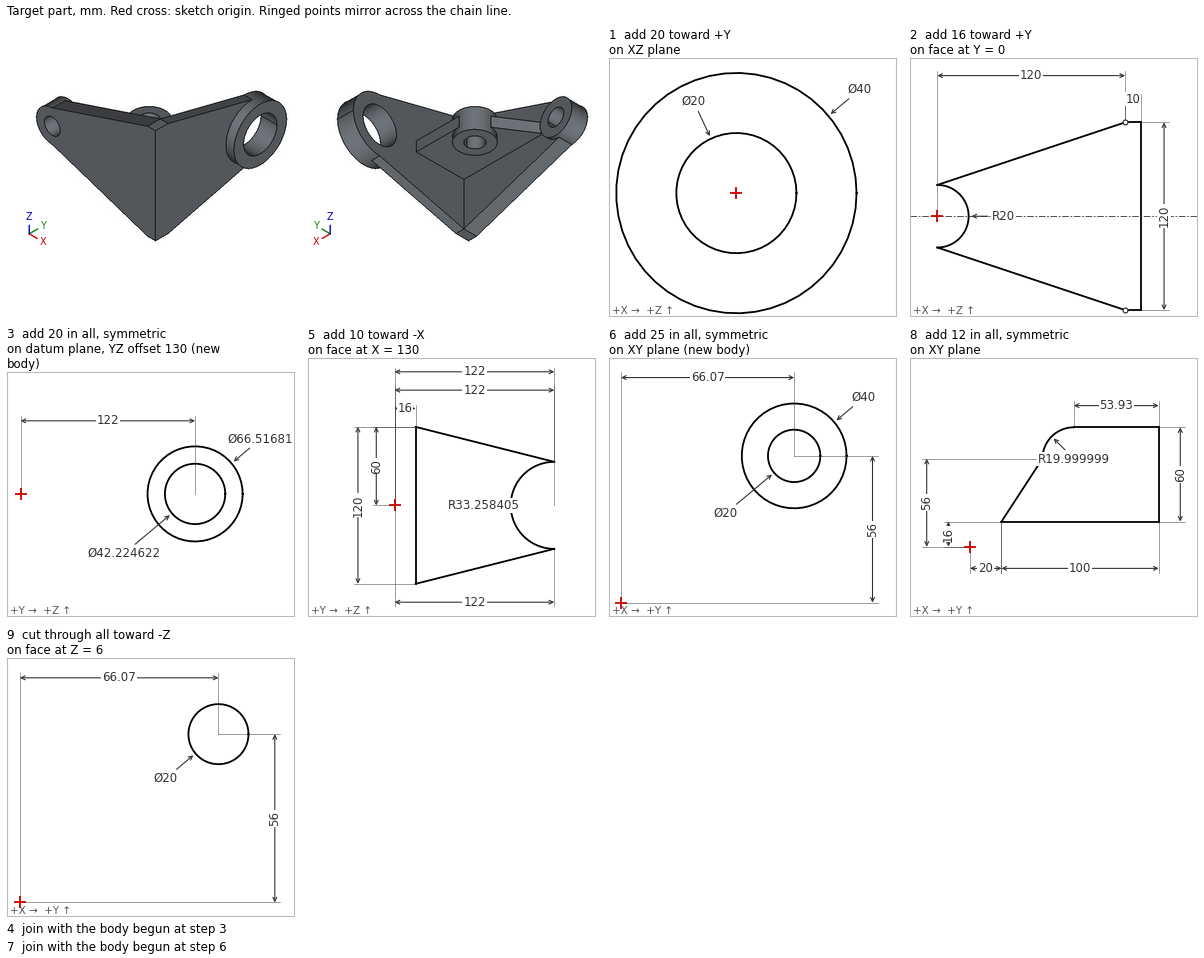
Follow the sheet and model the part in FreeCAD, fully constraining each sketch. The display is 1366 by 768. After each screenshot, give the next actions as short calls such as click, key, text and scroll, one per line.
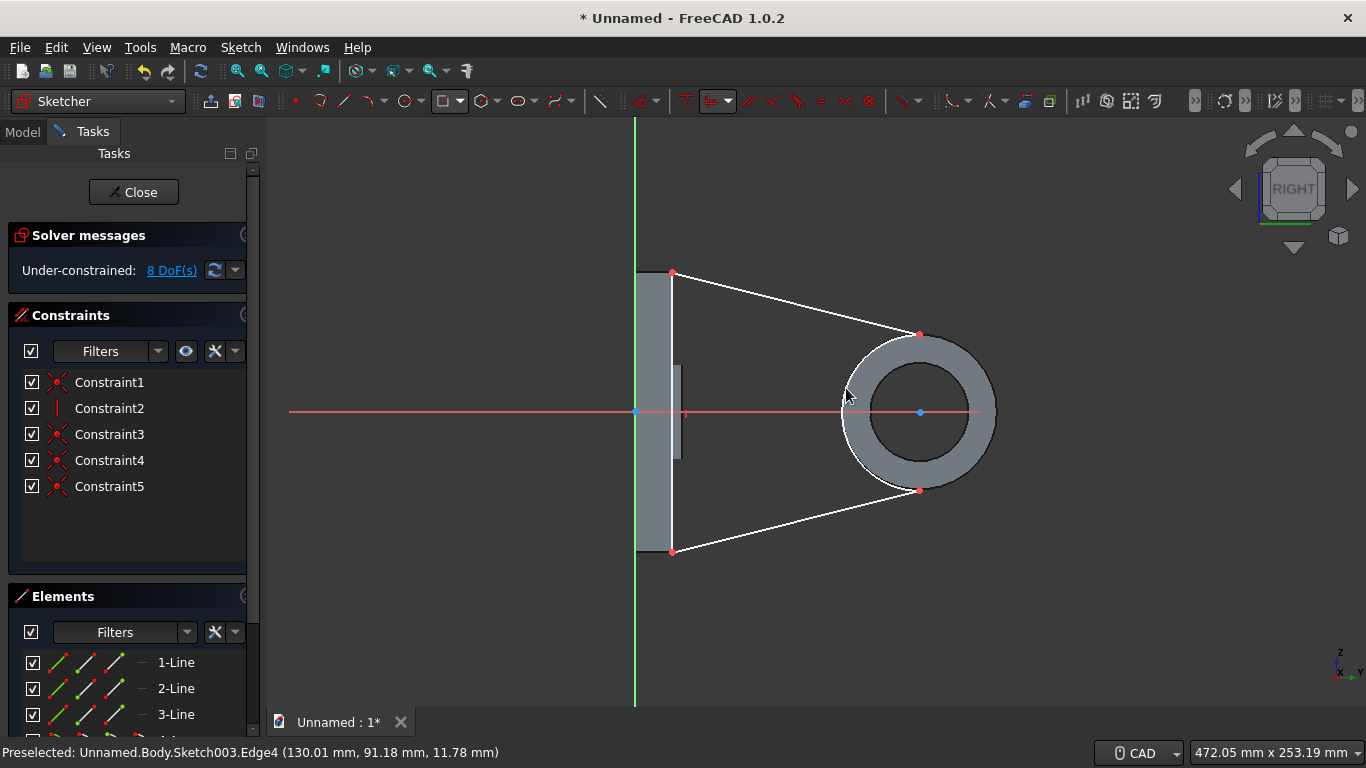
click(920, 413)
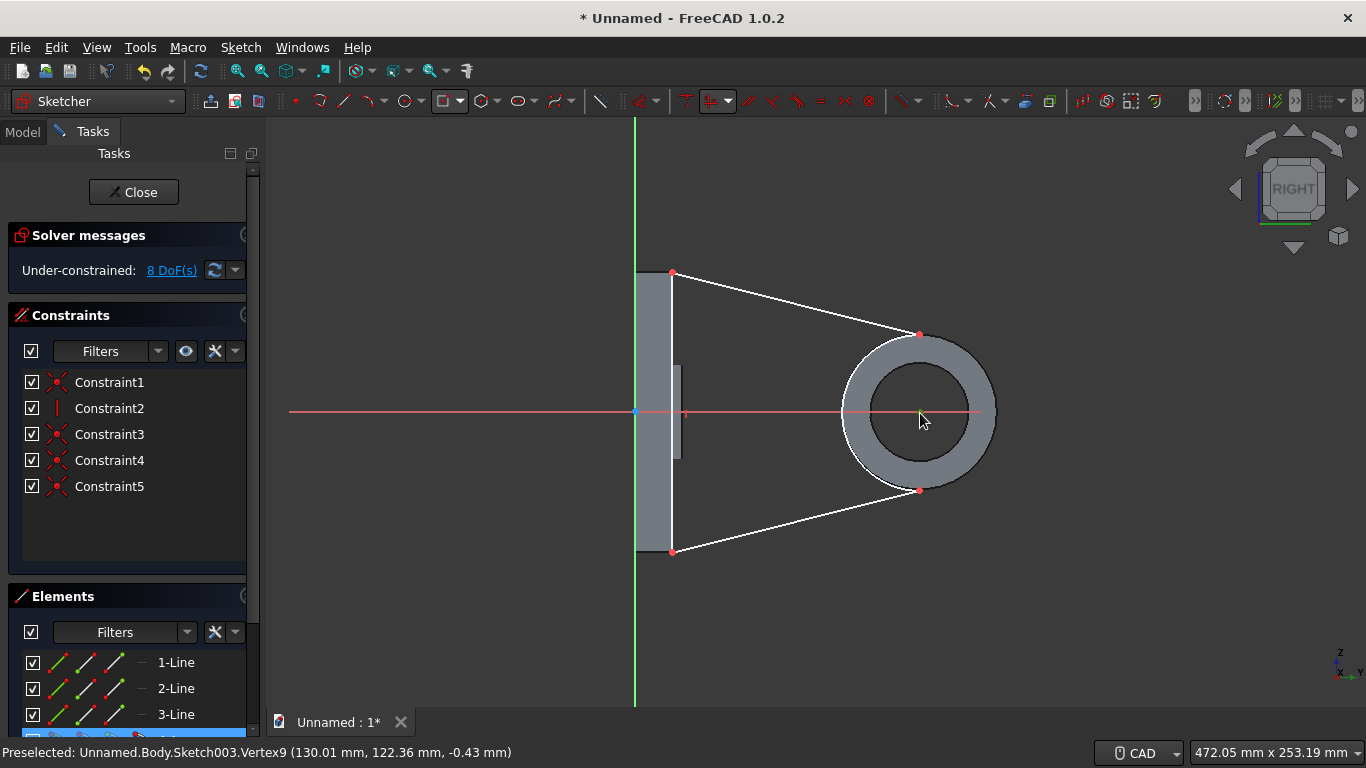
click(359, 412)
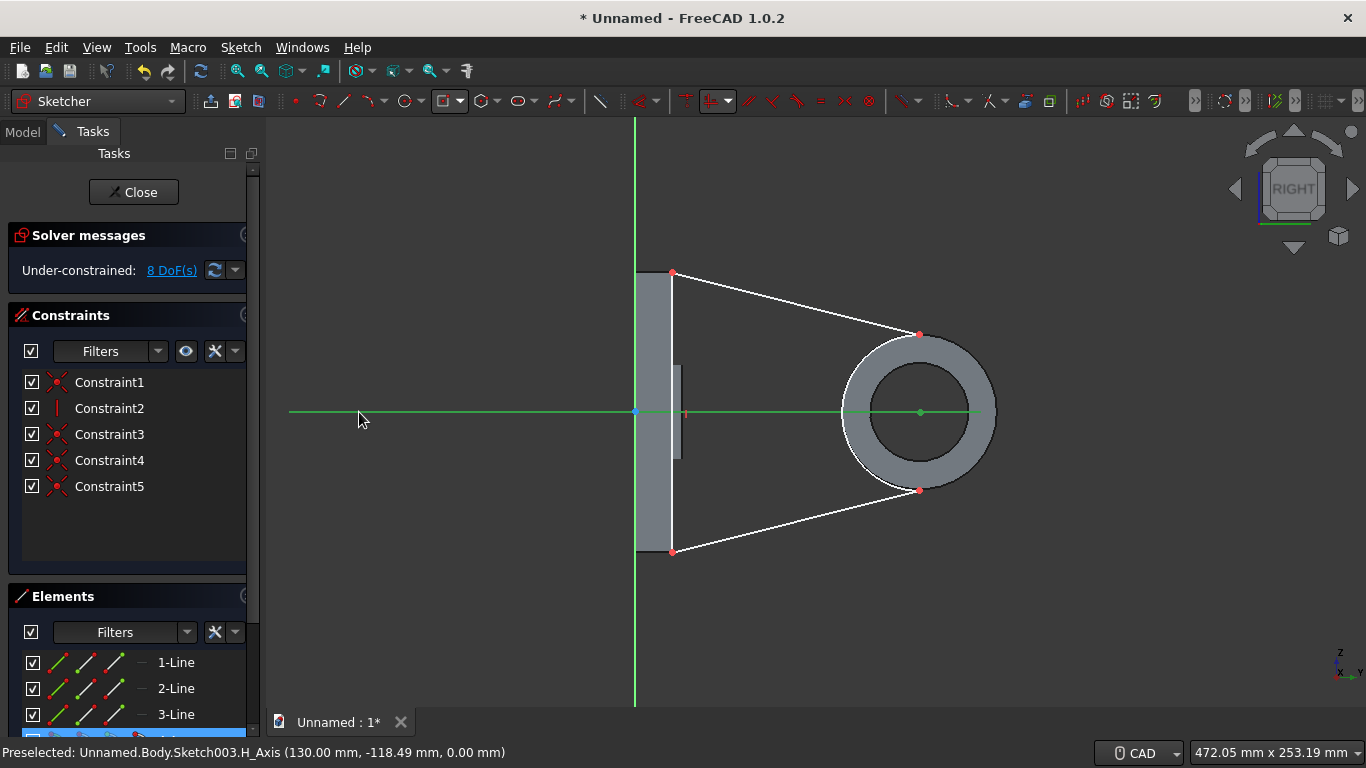
click(686, 102)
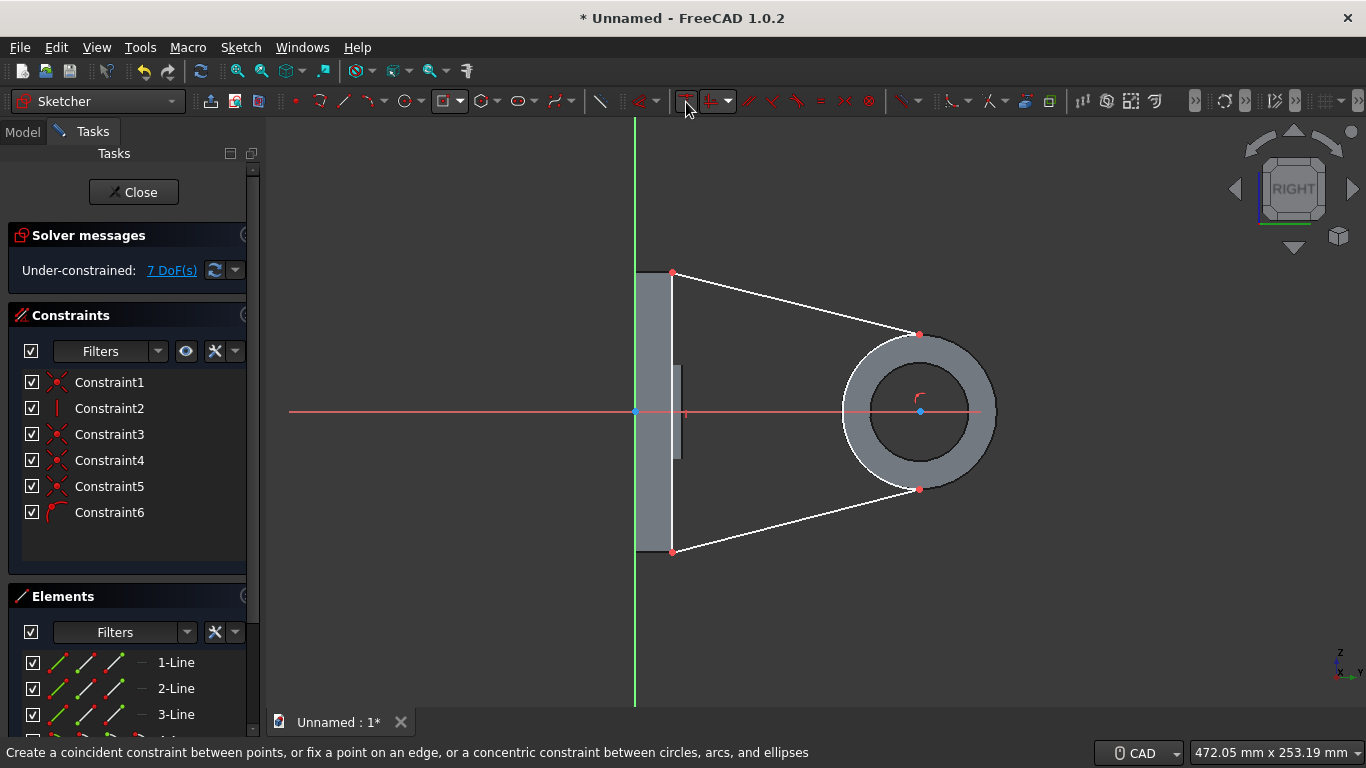
click(640, 102)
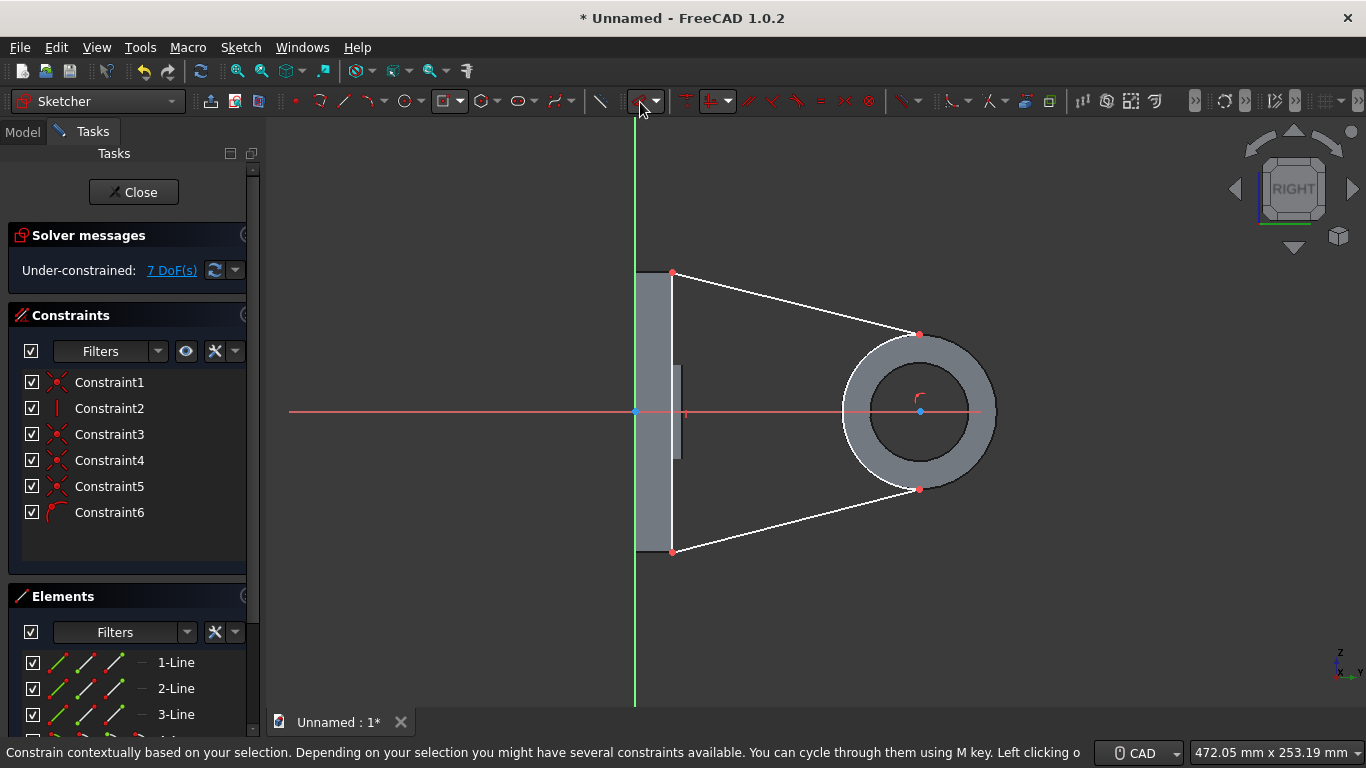
click(857, 367)
click(831, 348)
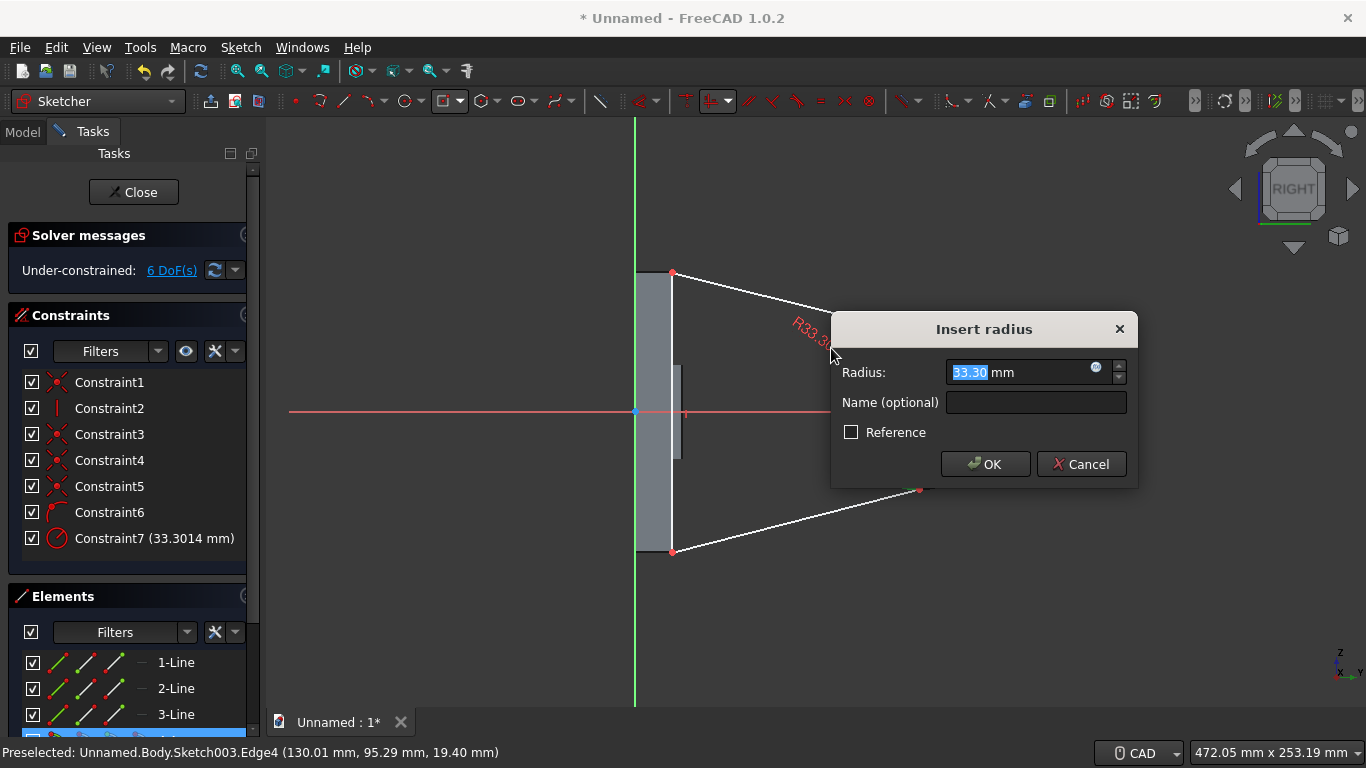
text(33.258405)
key(Return)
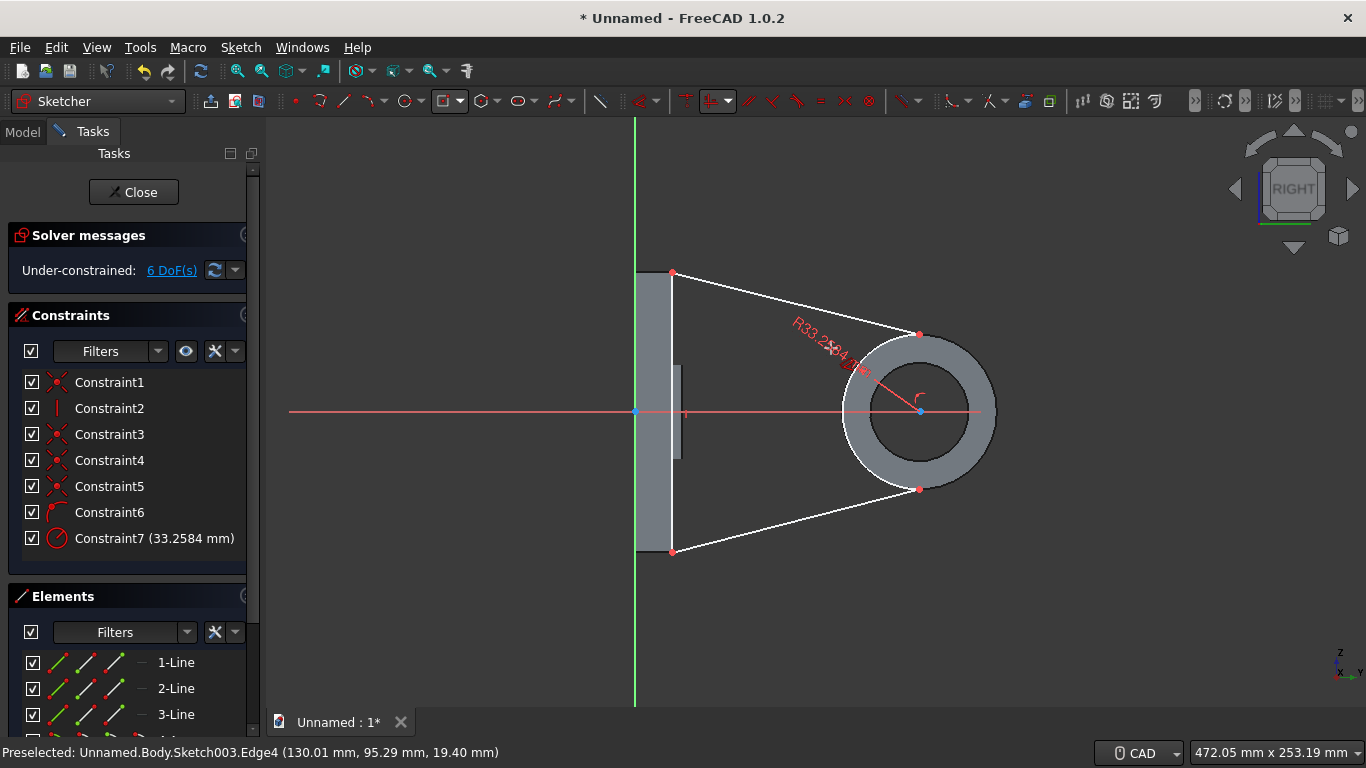
click(672, 357)
click(706, 349)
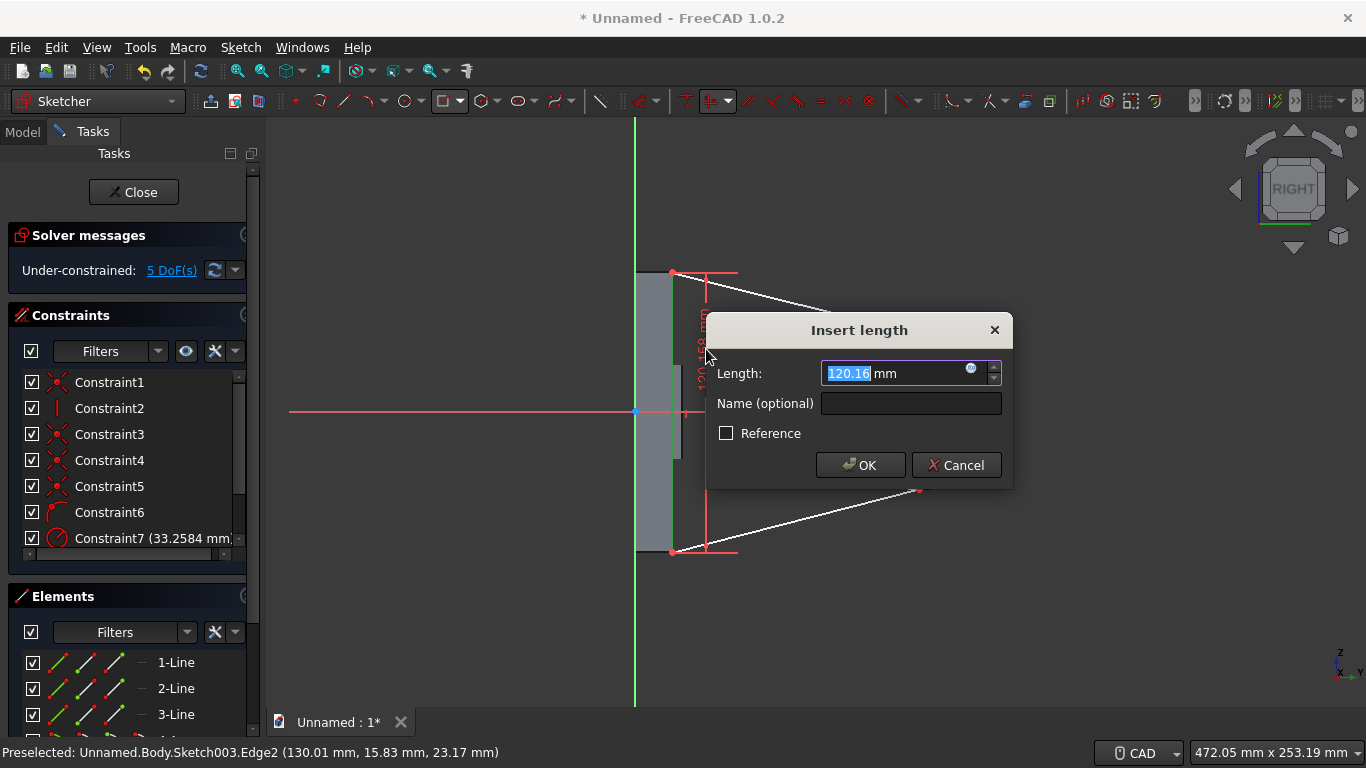
text(120)
key(Return)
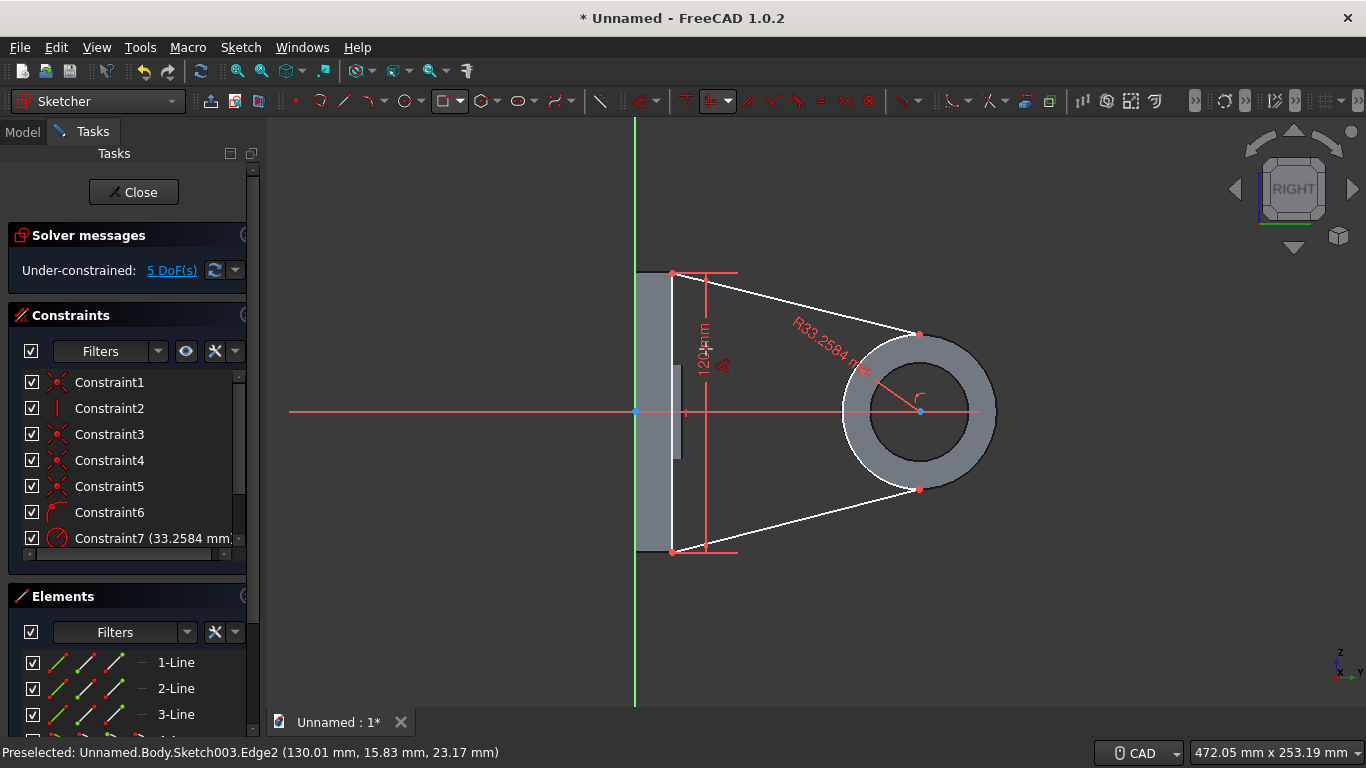
click(672, 273)
click(654, 239)